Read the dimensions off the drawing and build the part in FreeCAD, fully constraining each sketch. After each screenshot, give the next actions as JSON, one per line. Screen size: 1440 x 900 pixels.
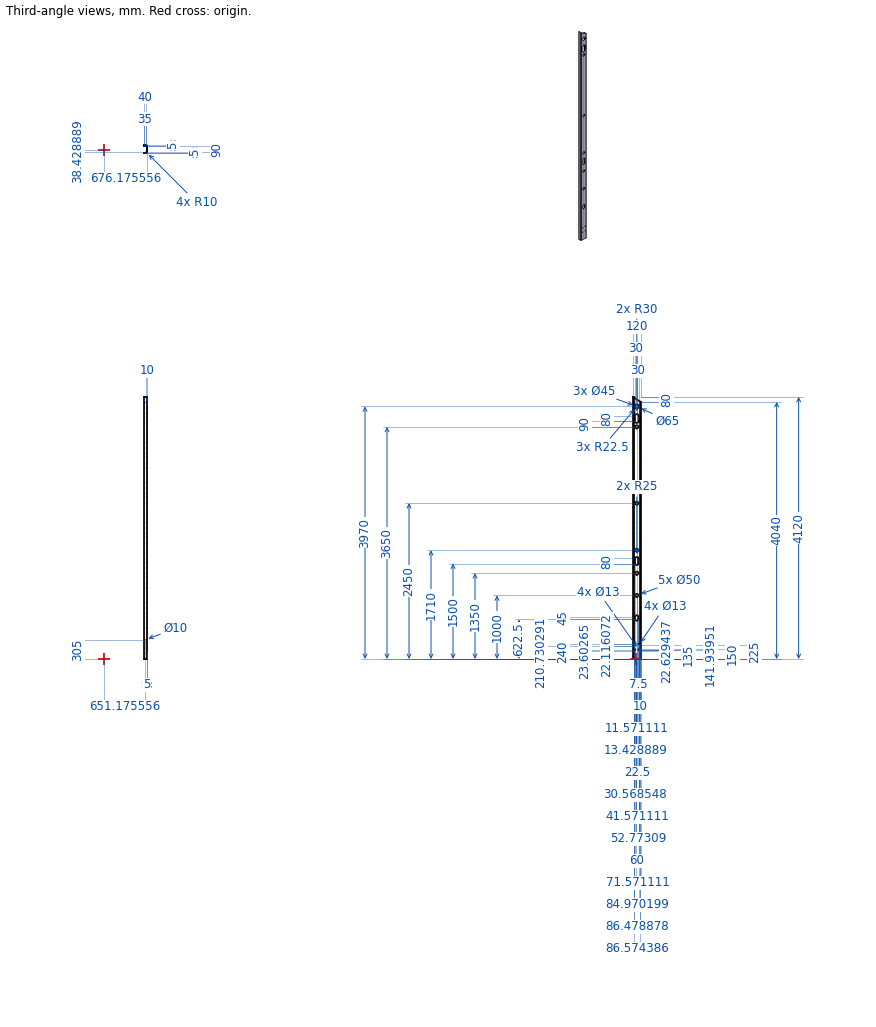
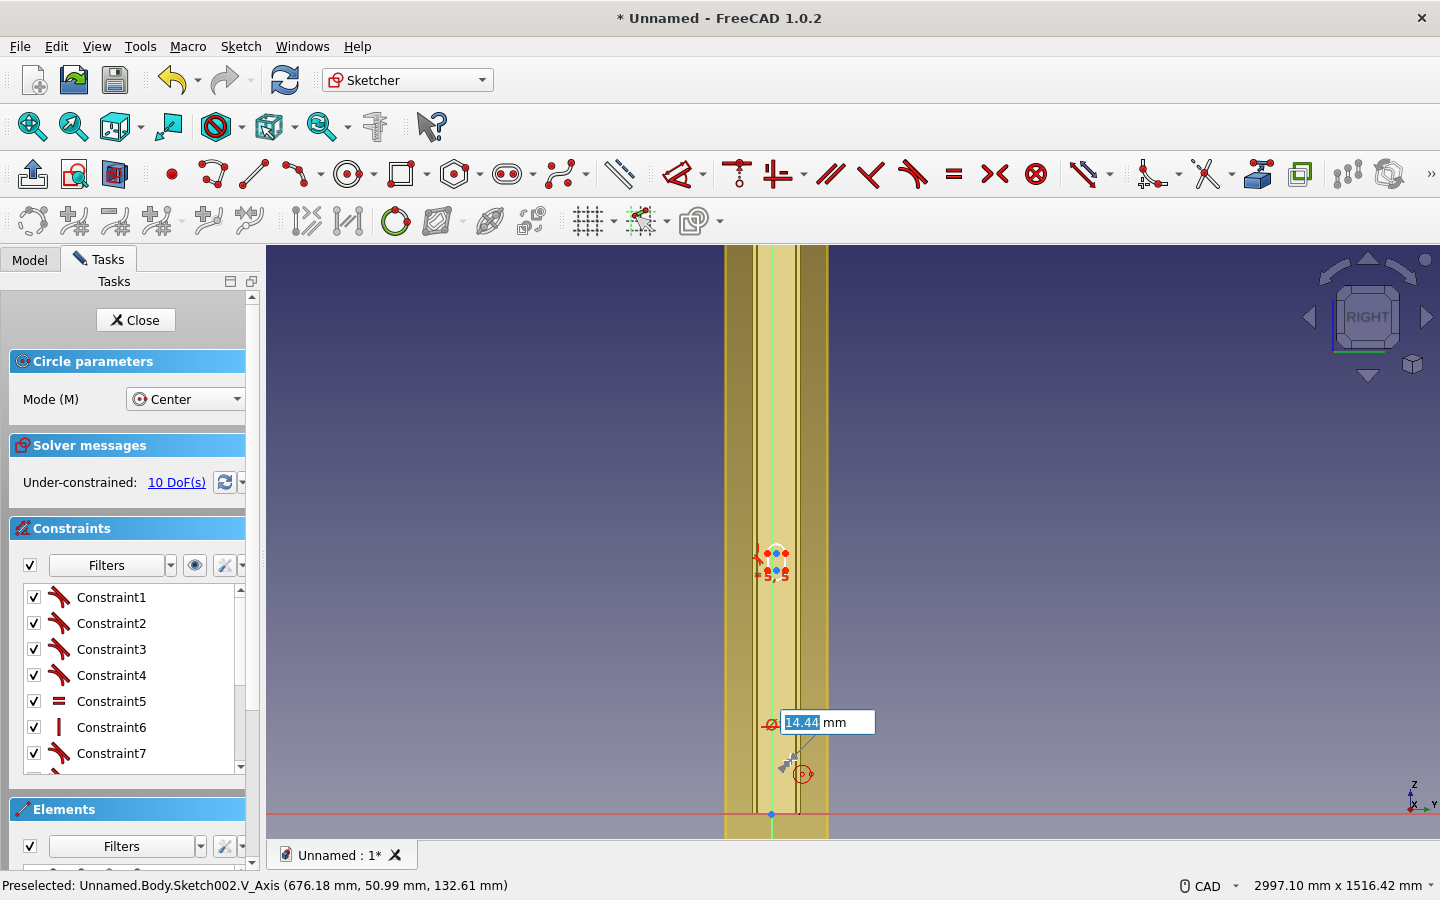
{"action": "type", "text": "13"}
{"action": "key", "text": "Return"}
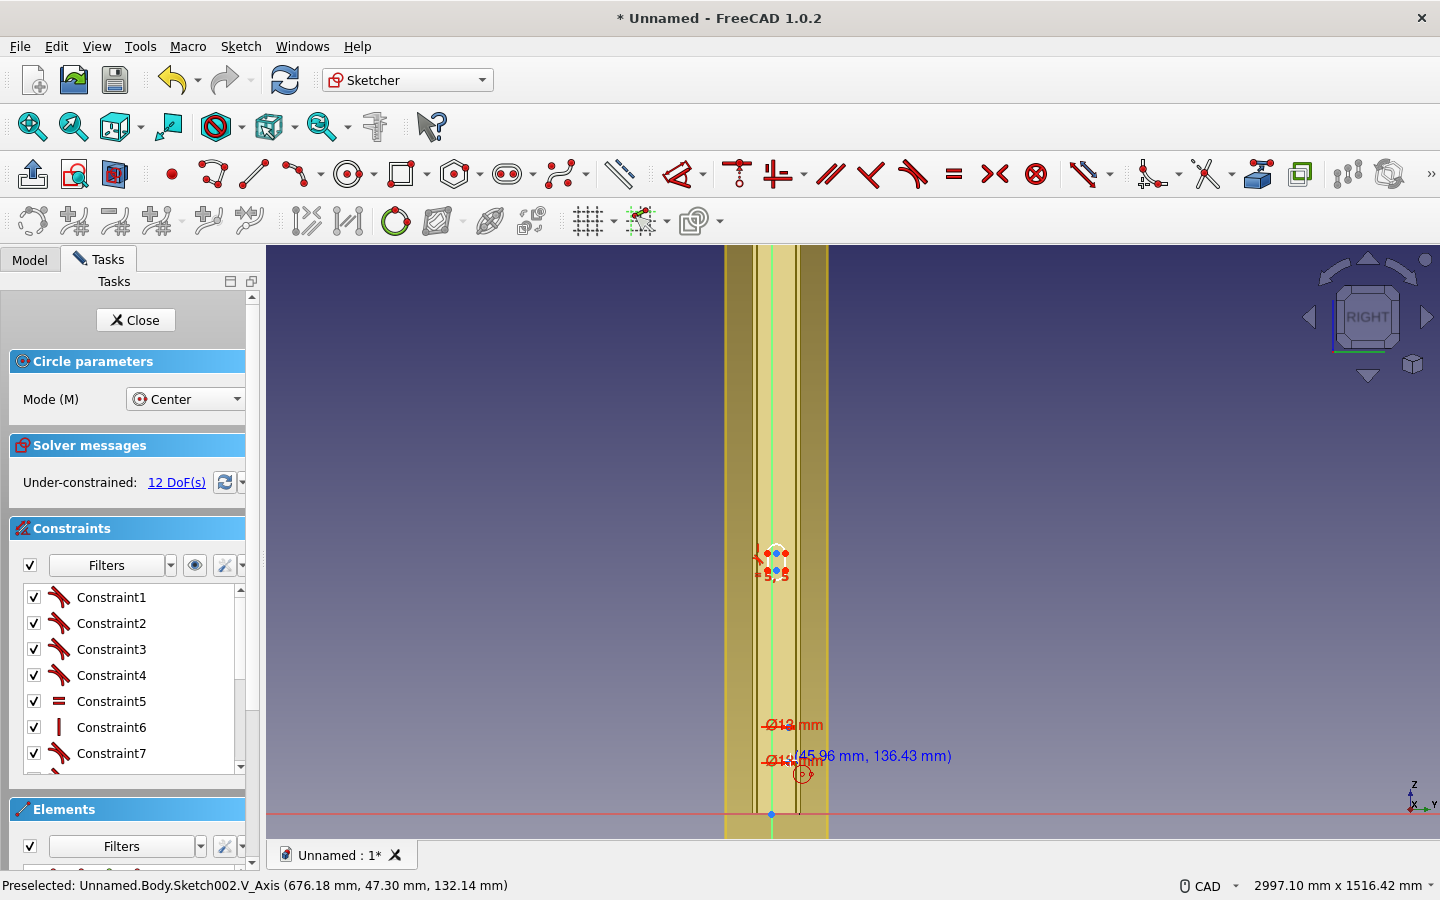
{"action": "scroll", "coordinate": [765, 762], "scroll_direction": "up", "scroll_amount": 11}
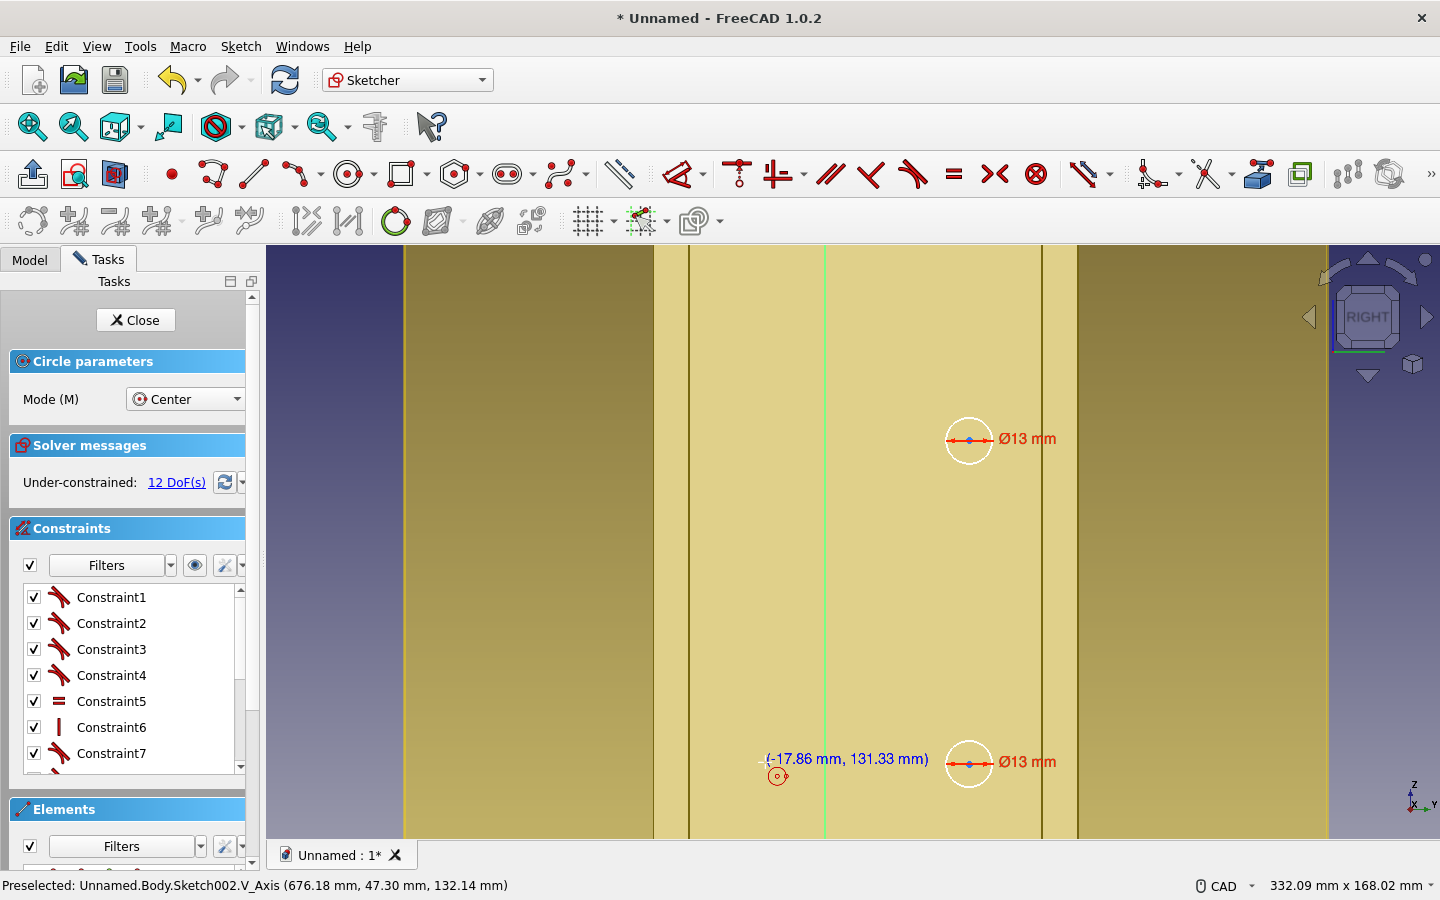
{"action": "scroll", "coordinate": [782, 762], "scroll_direction": "down", "scroll_amount": 17}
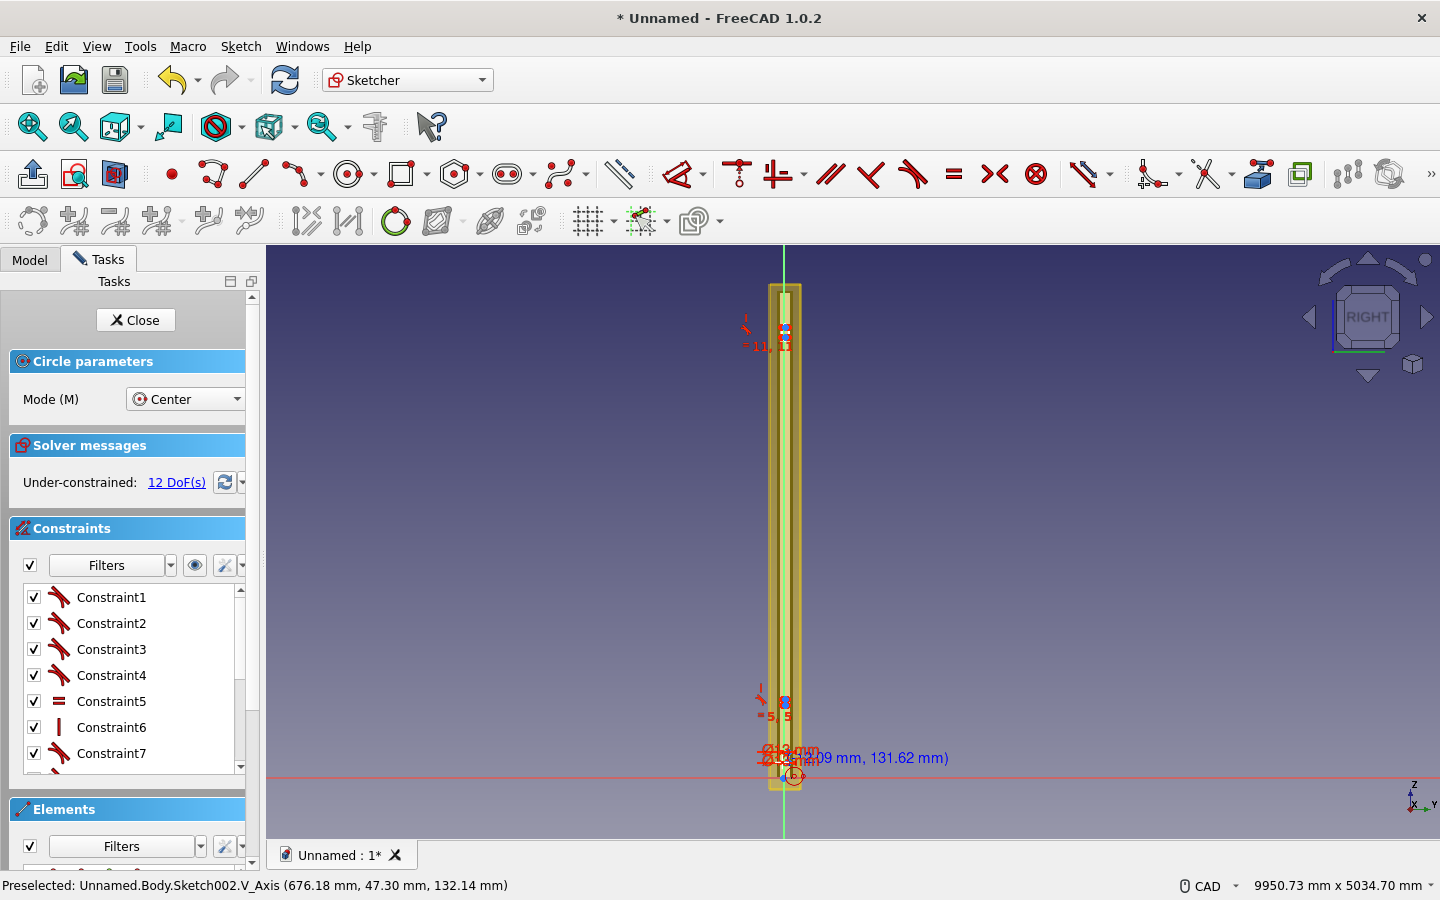
{"action": "scroll", "coordinate": [782, 762], "scroll_direction": "up", "scroll_amount": 10}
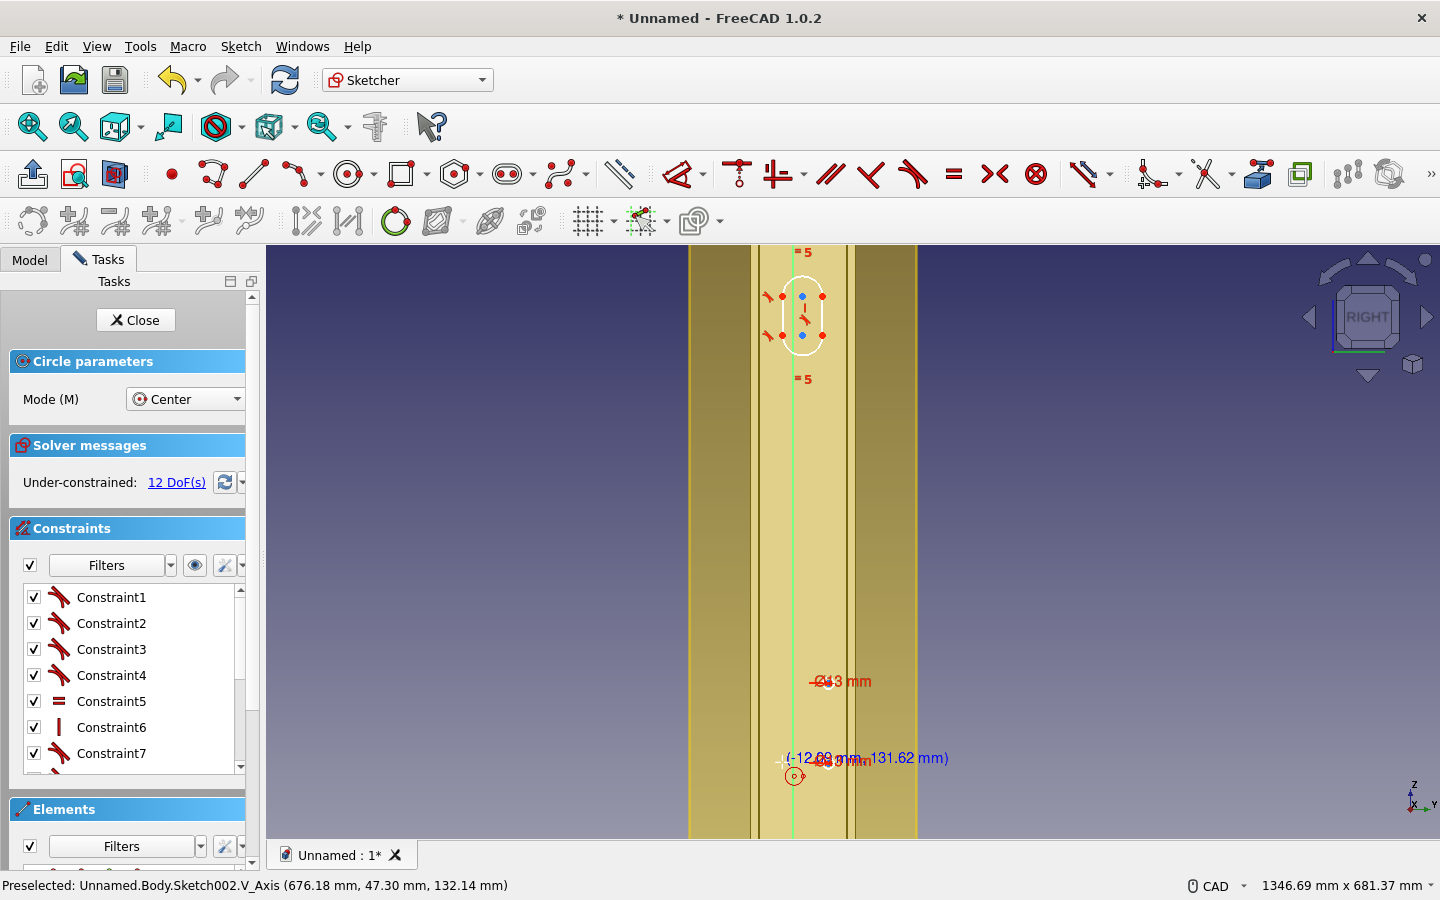
{"action": "left_click", "coordinate": [777, 760]}
{"action": "mouse_move", "coordinate": [773, 756]}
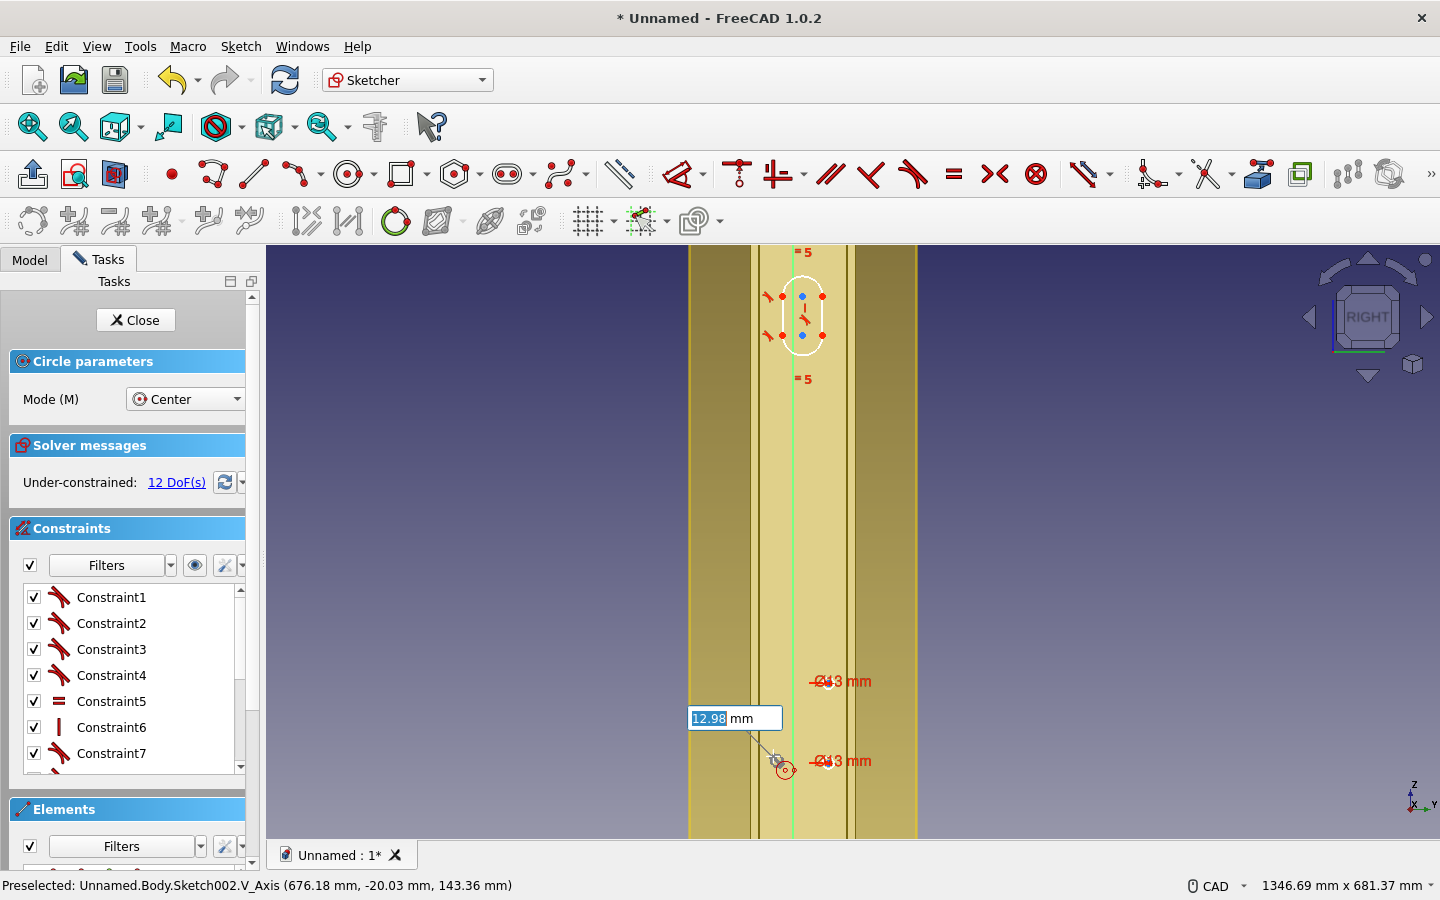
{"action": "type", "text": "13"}
{"action": "key", "text": "Return"}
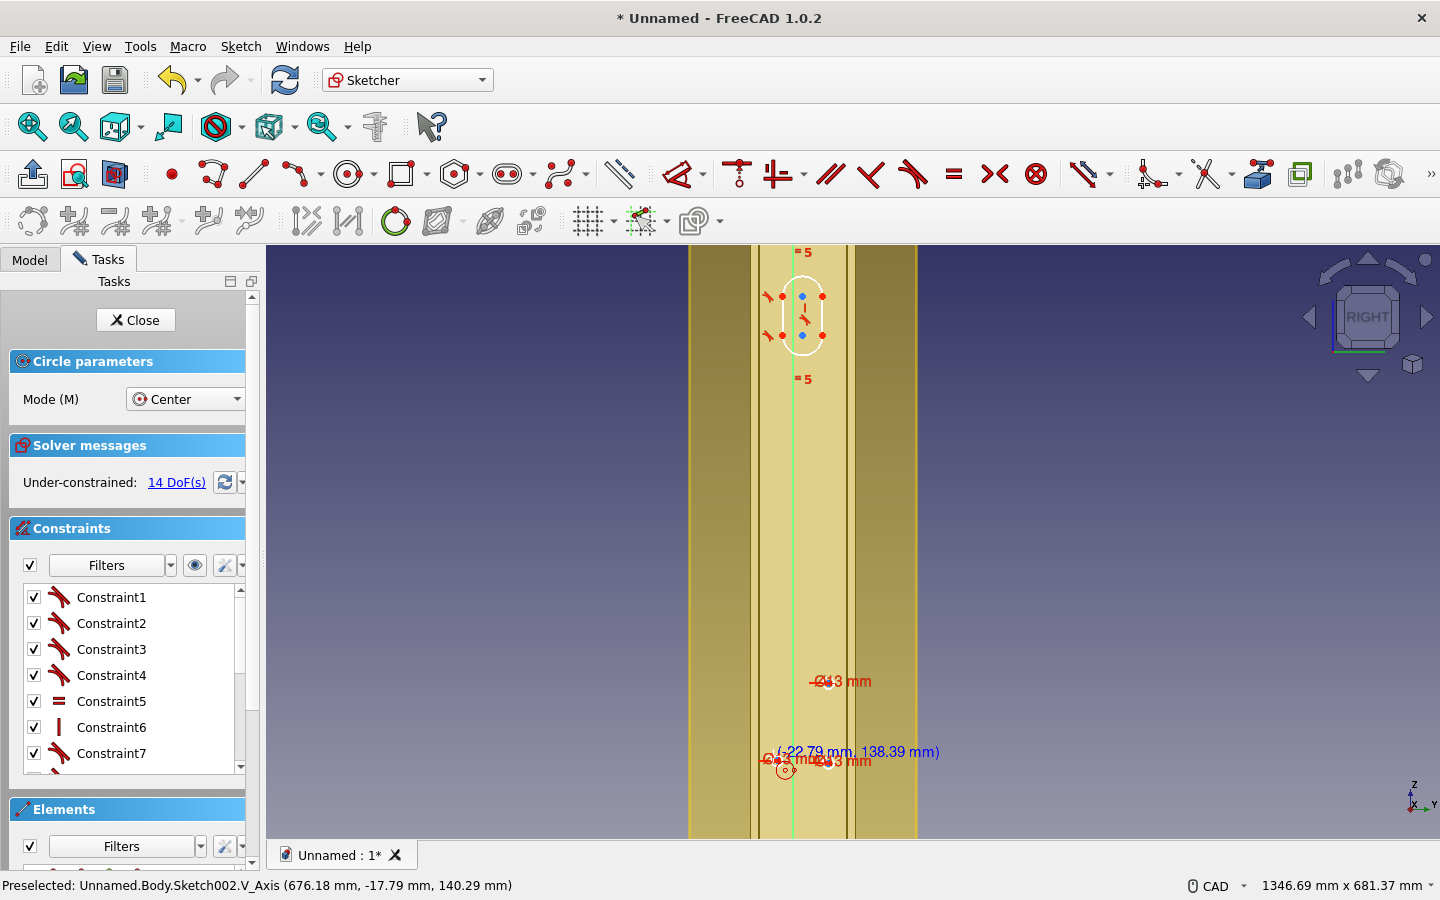
{"action": "scroll", "coordinate": [777, 681], "scroll_direction": "up", "scroll_amount": 7}